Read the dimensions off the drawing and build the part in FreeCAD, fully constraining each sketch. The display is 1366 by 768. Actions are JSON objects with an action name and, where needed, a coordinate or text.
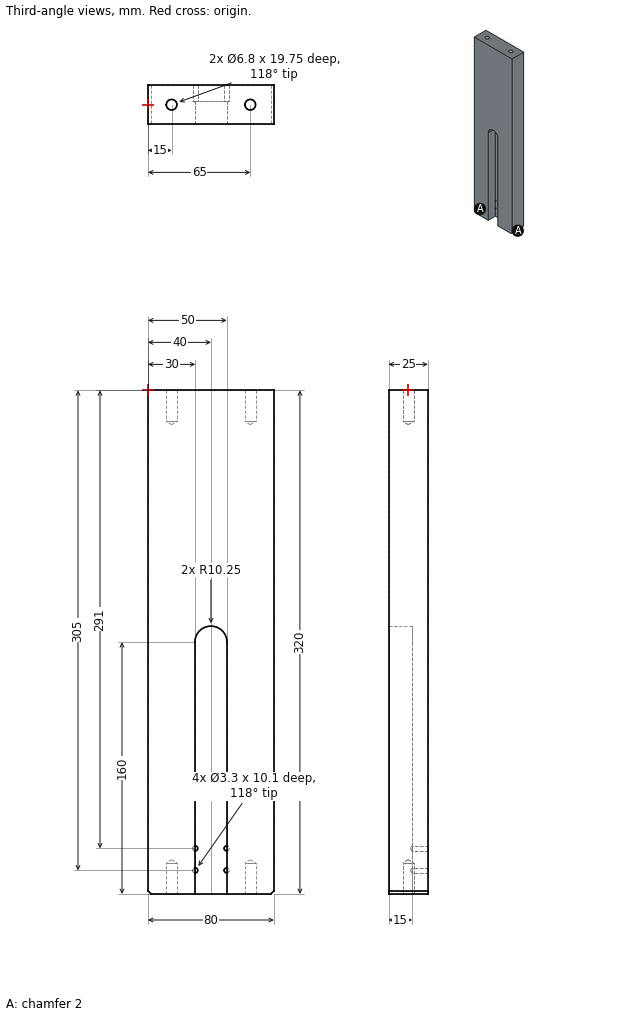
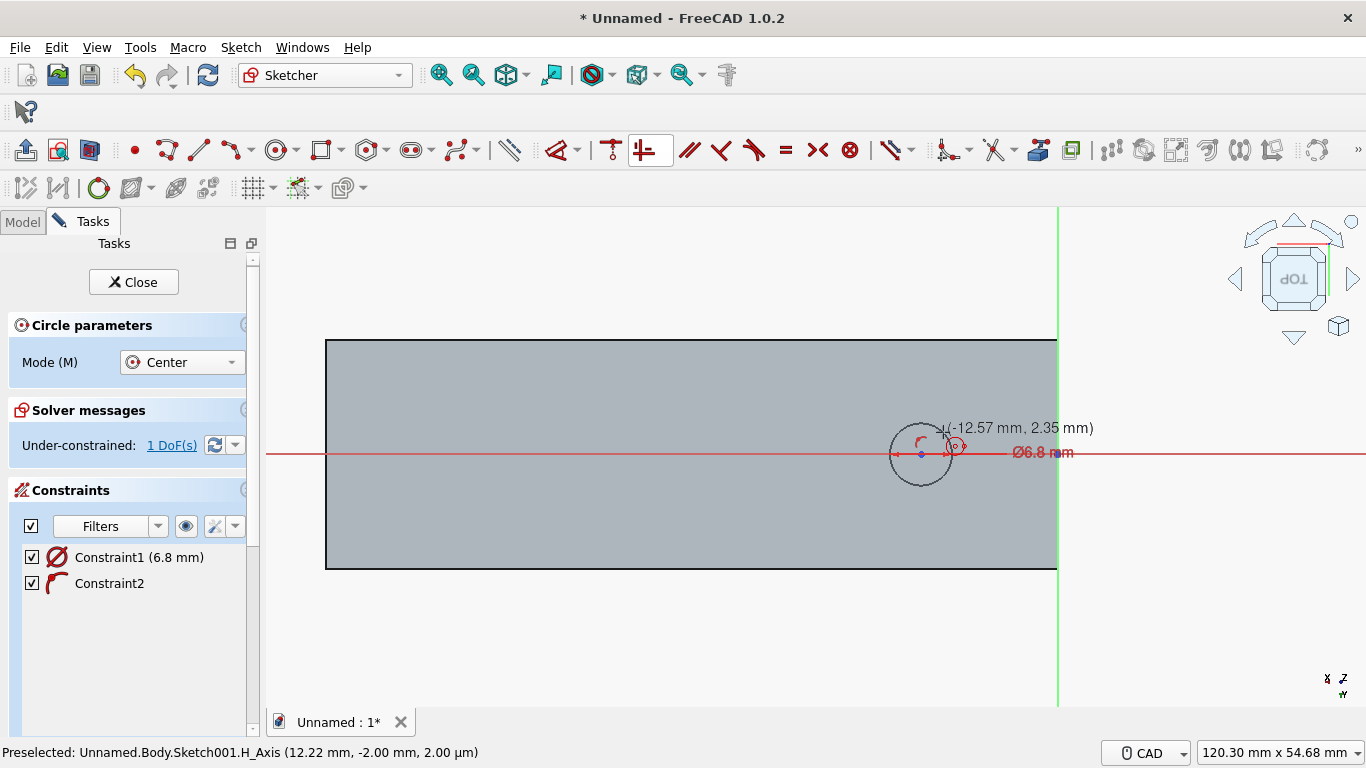
{"action": "left_click", "coordinate": [464, 454]}
{"action": "mouse_move", "coordinate": [486, 432]}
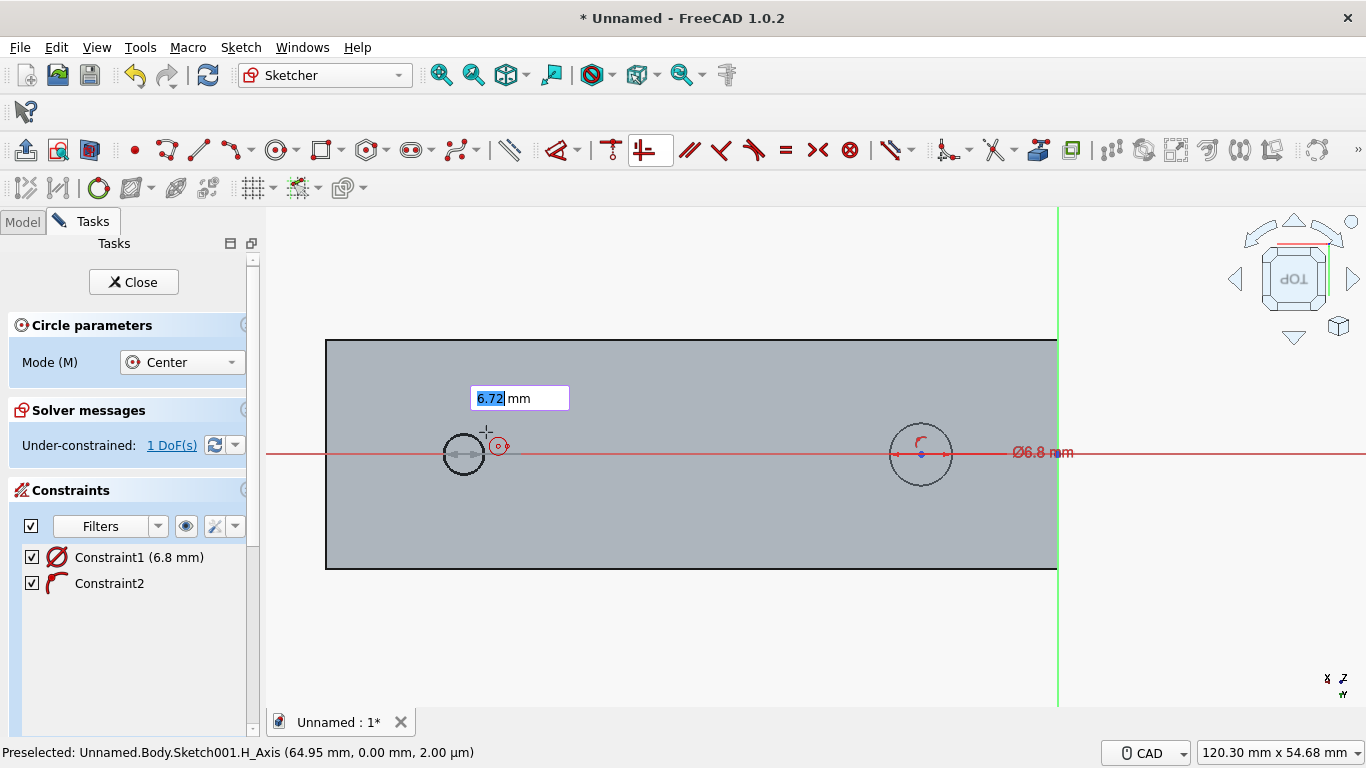
{"action": "type", "text": "6.8"}
{"action": "key", "text": "Return"}
{"action": "key", "text": "Escape"}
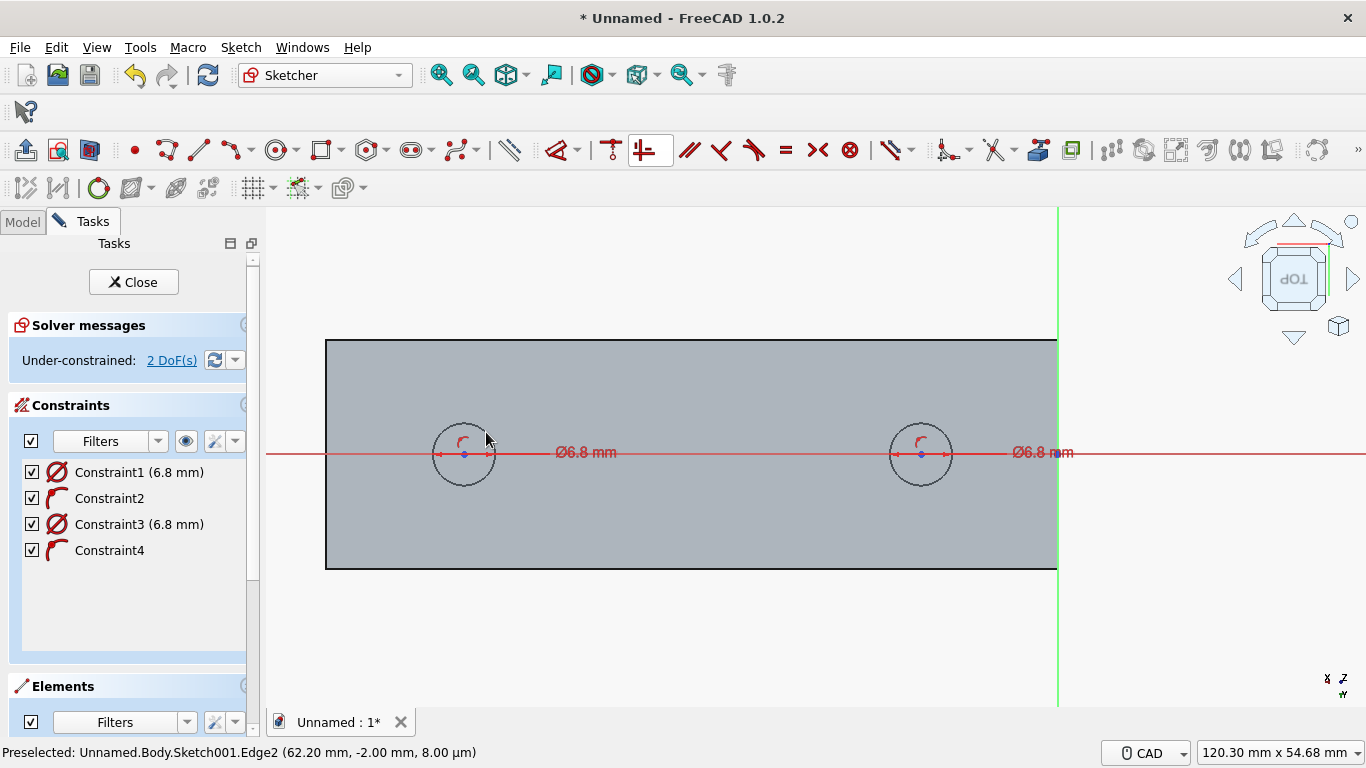
{"action": "left_click", "coordinate": [556, 150]}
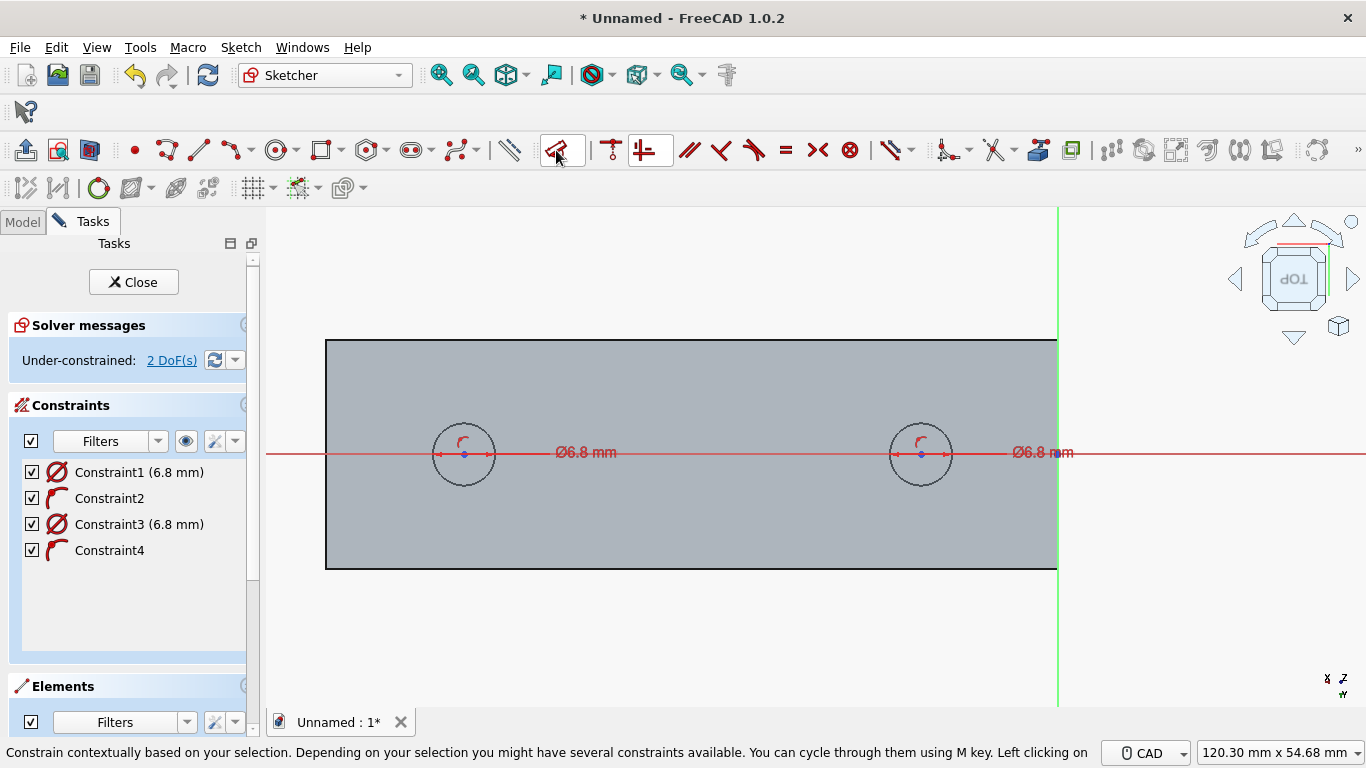
{"action": "left_click", "coordinate": [921, 454]}
{"action": "left_click", "coordinate": [989, 488]}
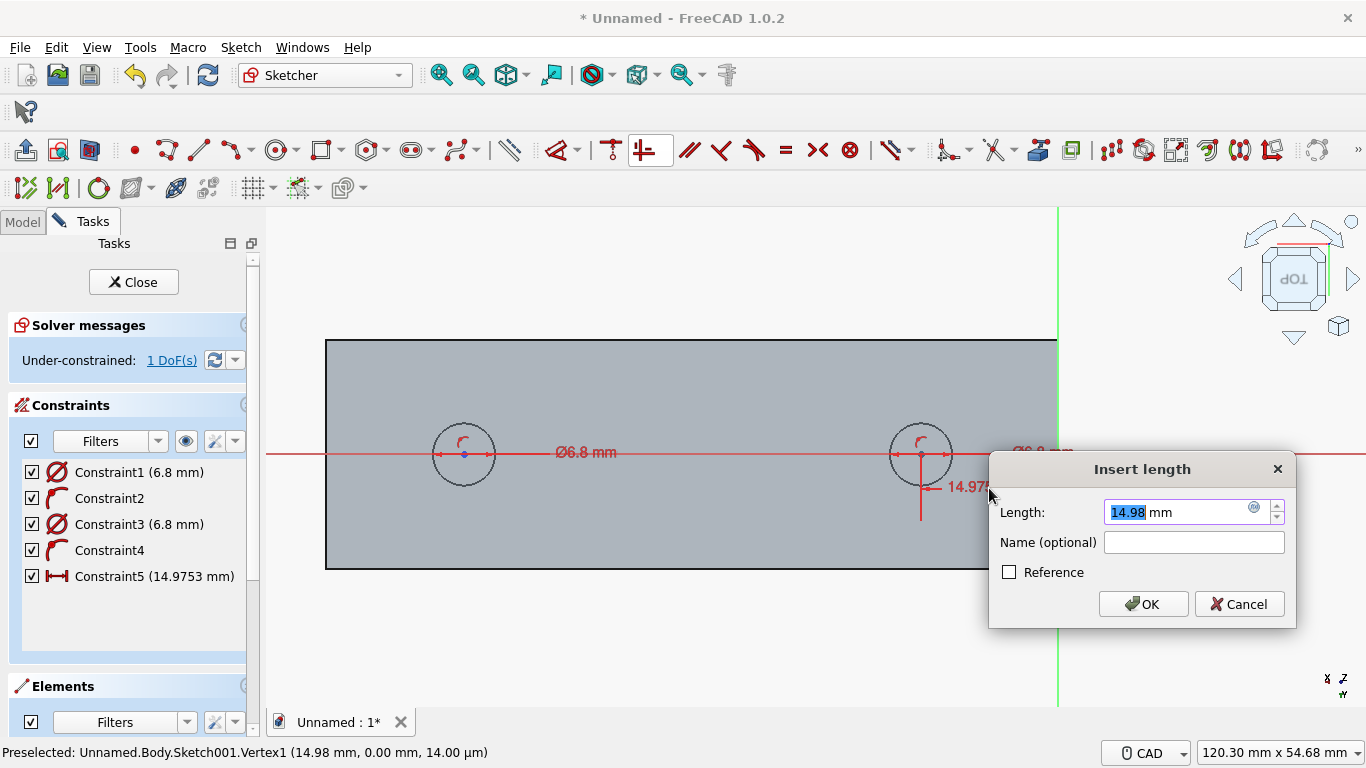
{"action": "type", "text": "15"}
{"action": "key", "text": "Return"}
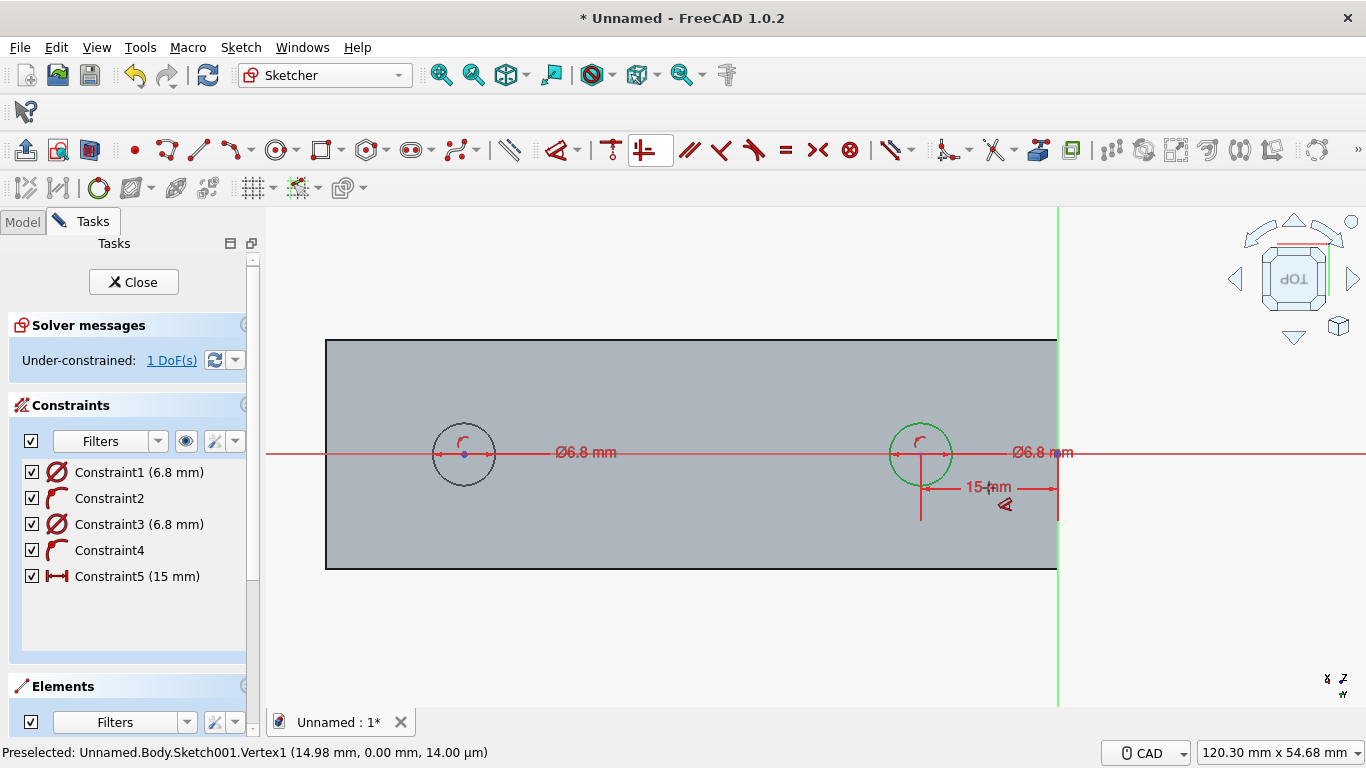
{"action": "left_click", "coordinate": [464, 454]}
{"action": "left_click", "coordinate": [761, 488]}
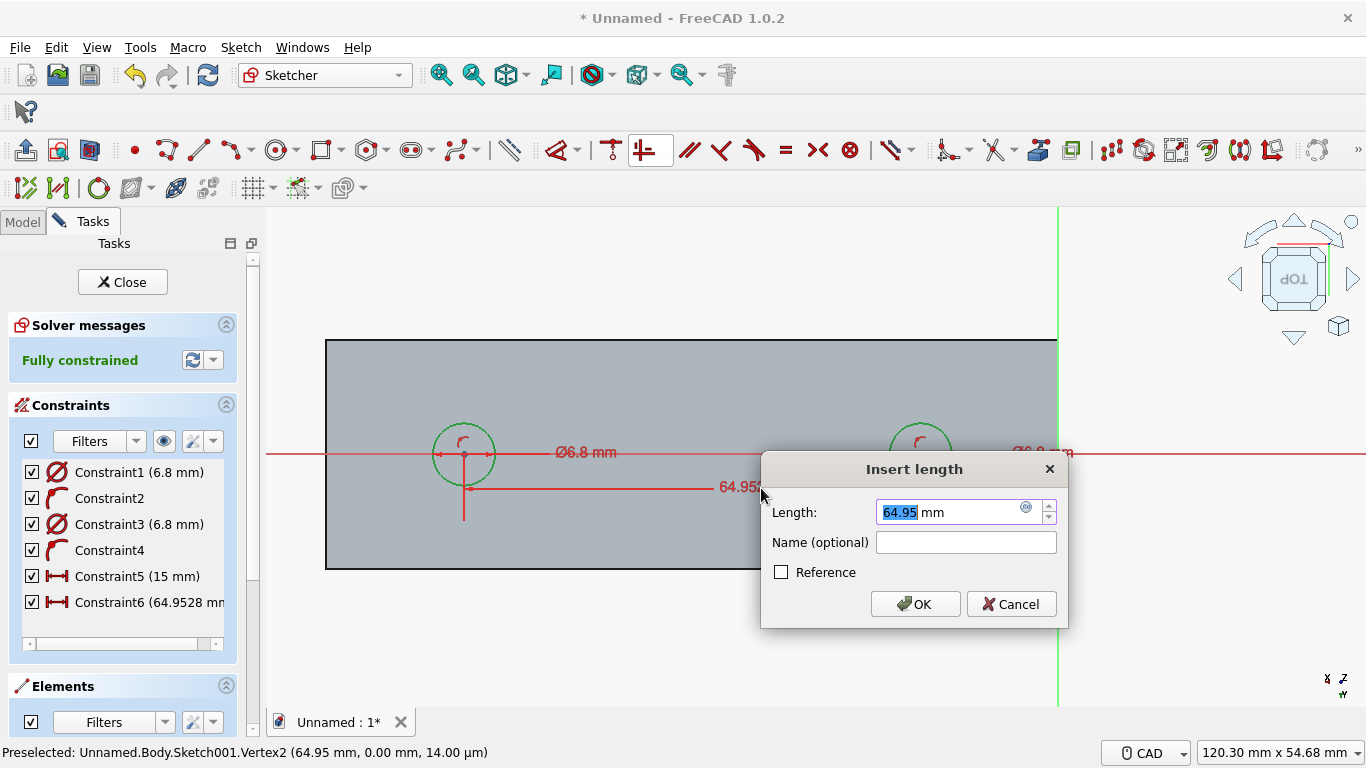
{"action": "type", "text": "65"}
{"action": "key", "text": "Return"}
{"action": "key", "text": "Escape"}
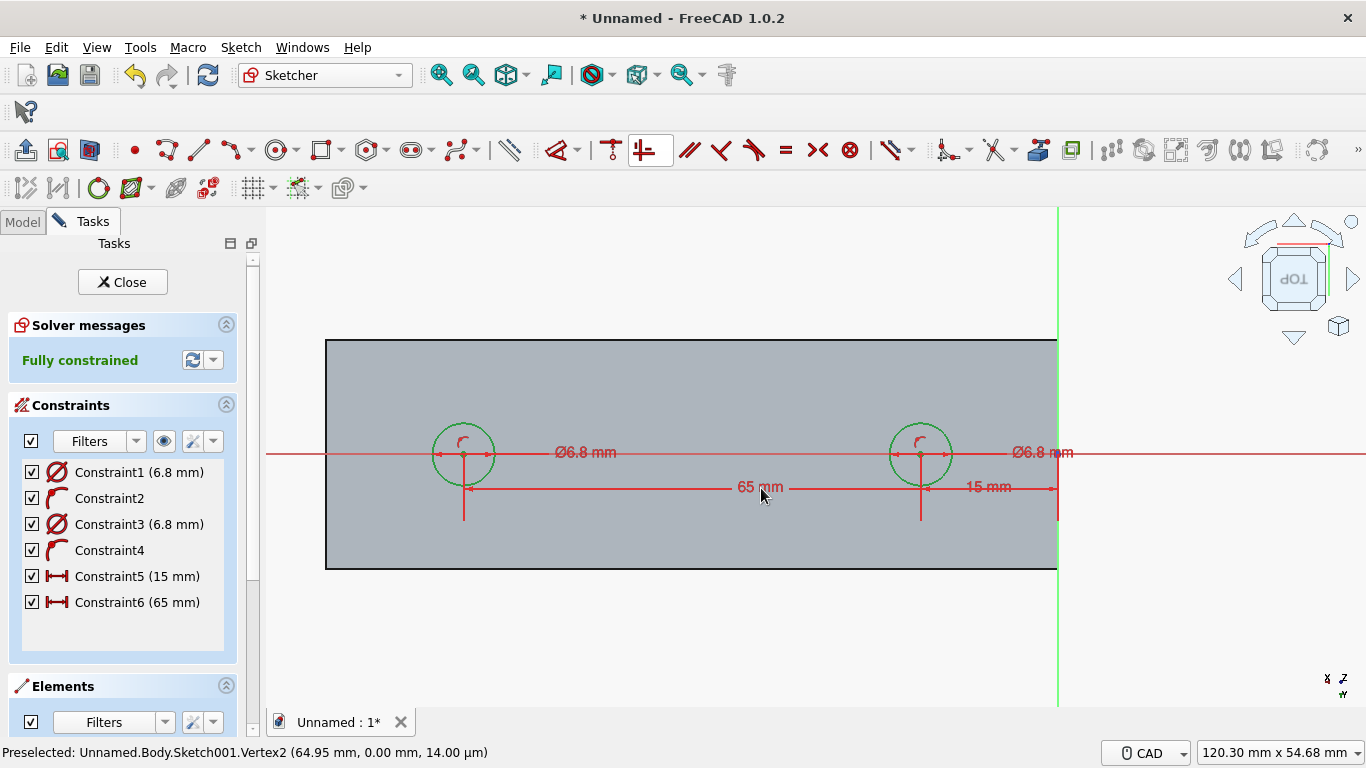
{"action": "left_click", "coordinate": [123, 282]}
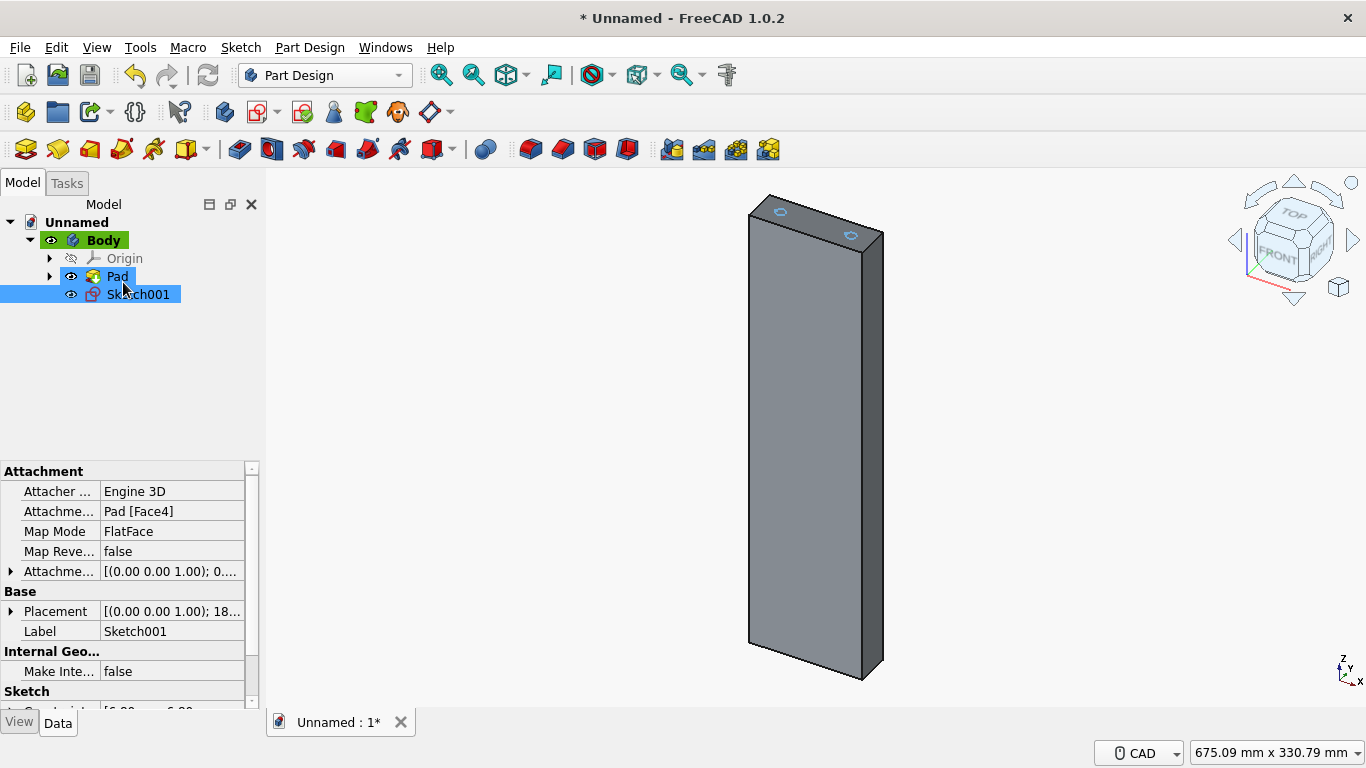
{"action": "left_click", "coordinate": [272, 150]}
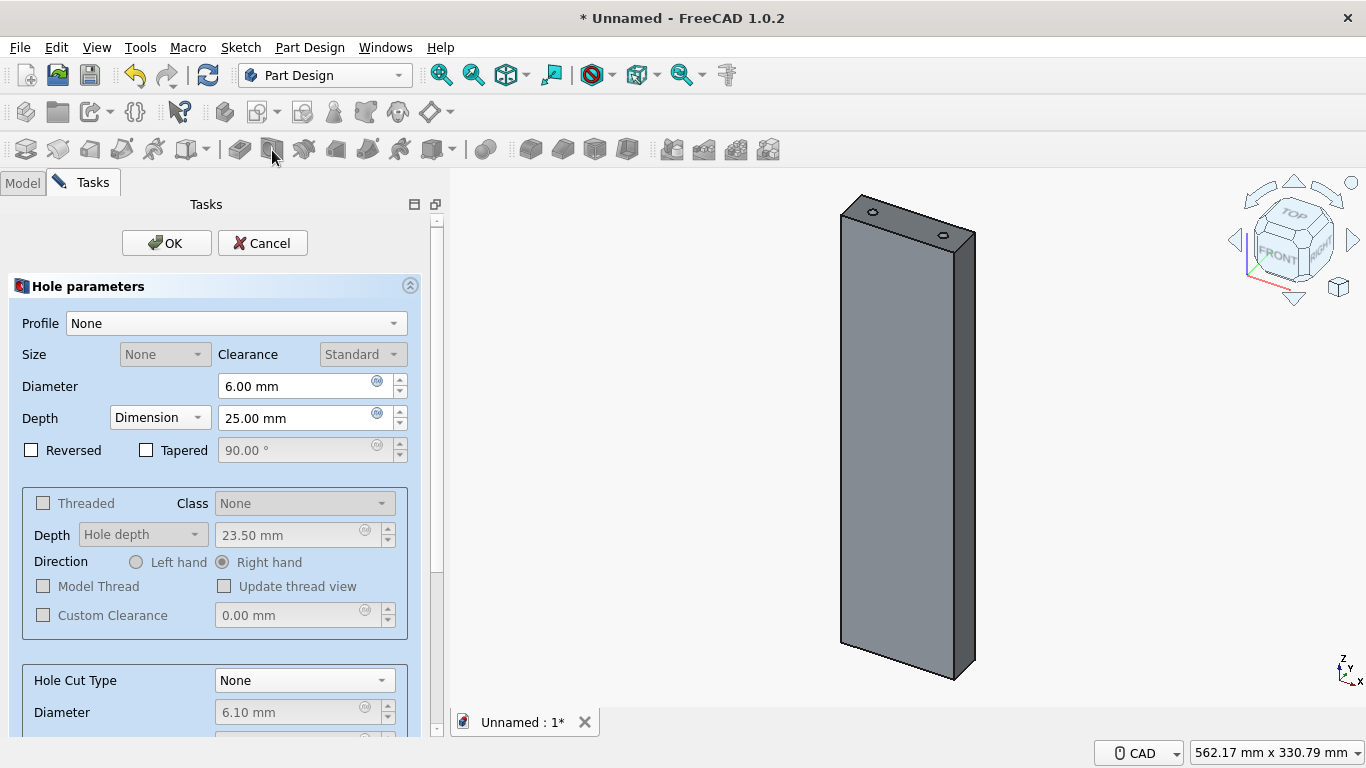
{"action": "triple_click", "coordinate": [305, 386]}